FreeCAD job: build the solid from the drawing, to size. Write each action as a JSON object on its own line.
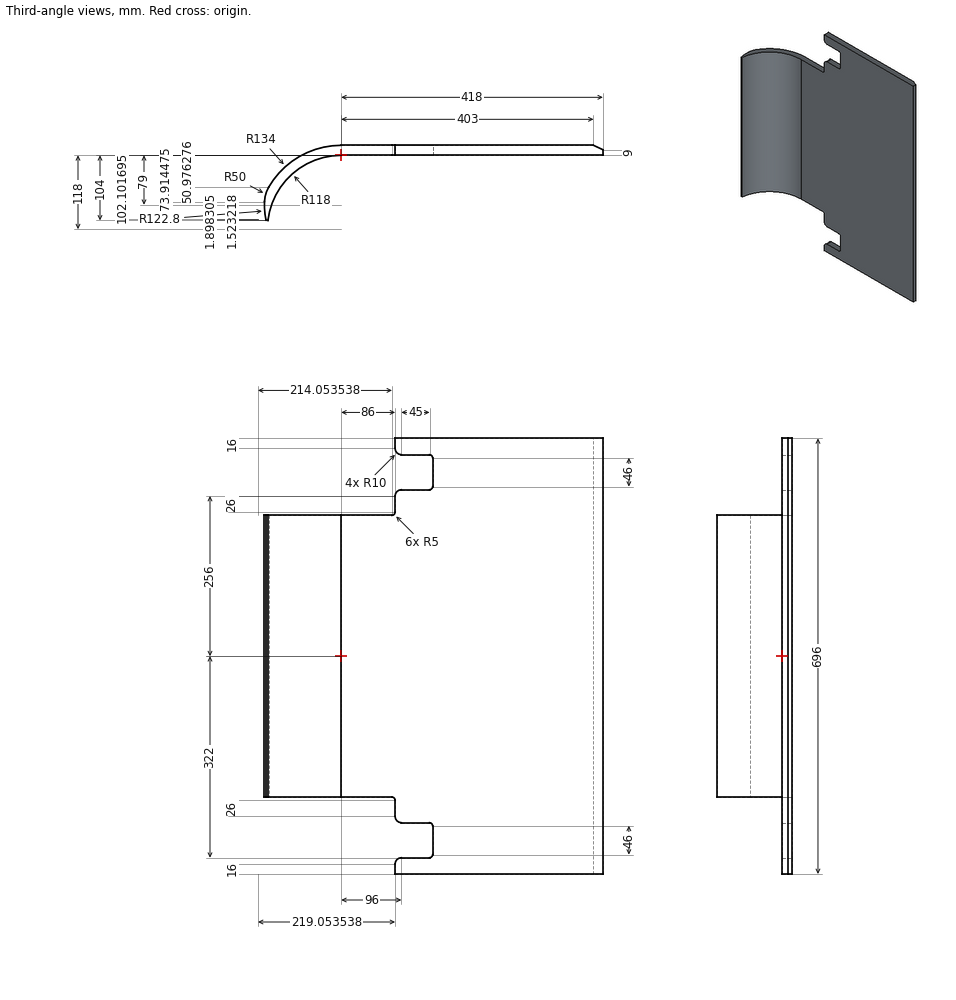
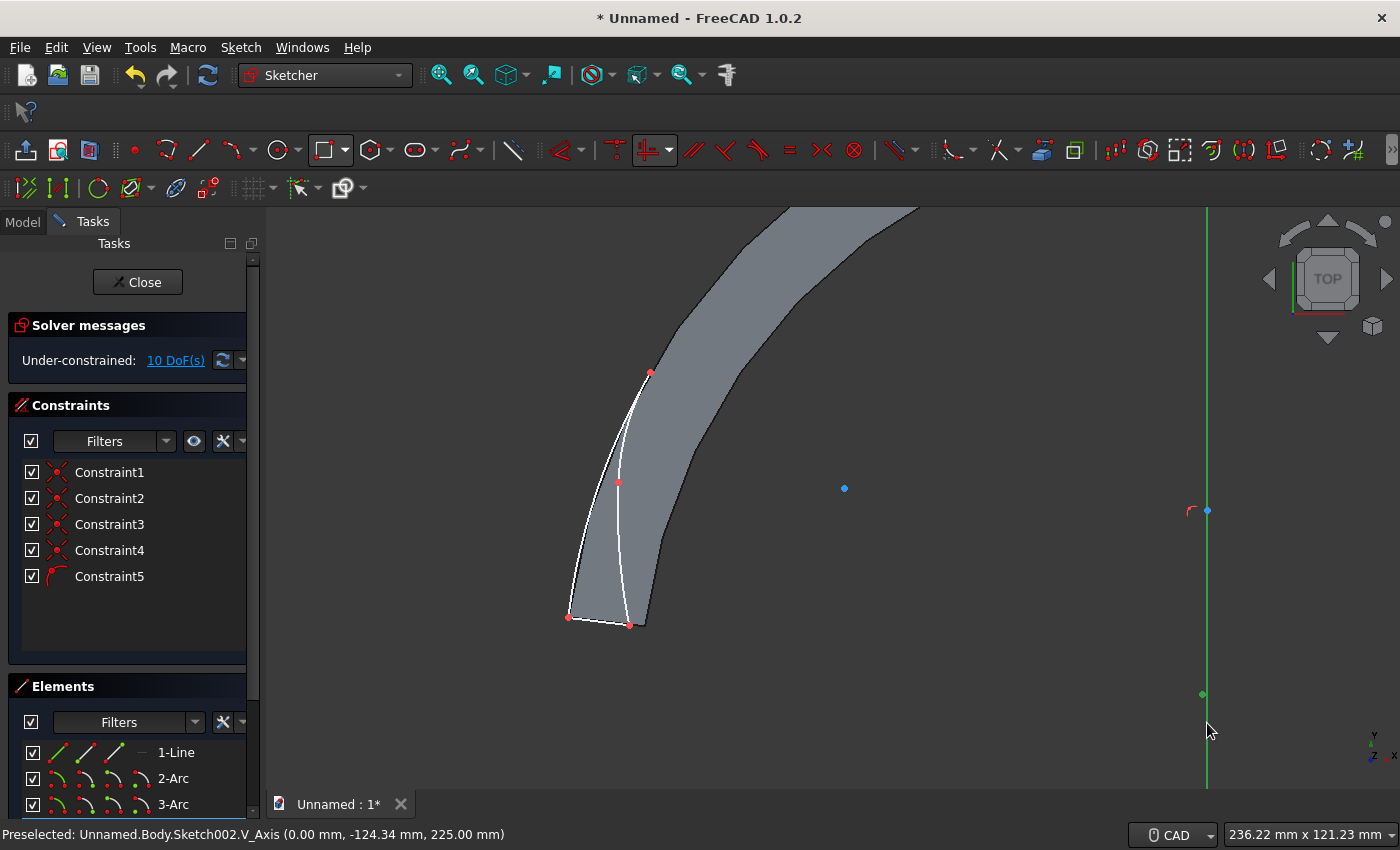
{"action": "left_click", "coordinate": [616, 150]}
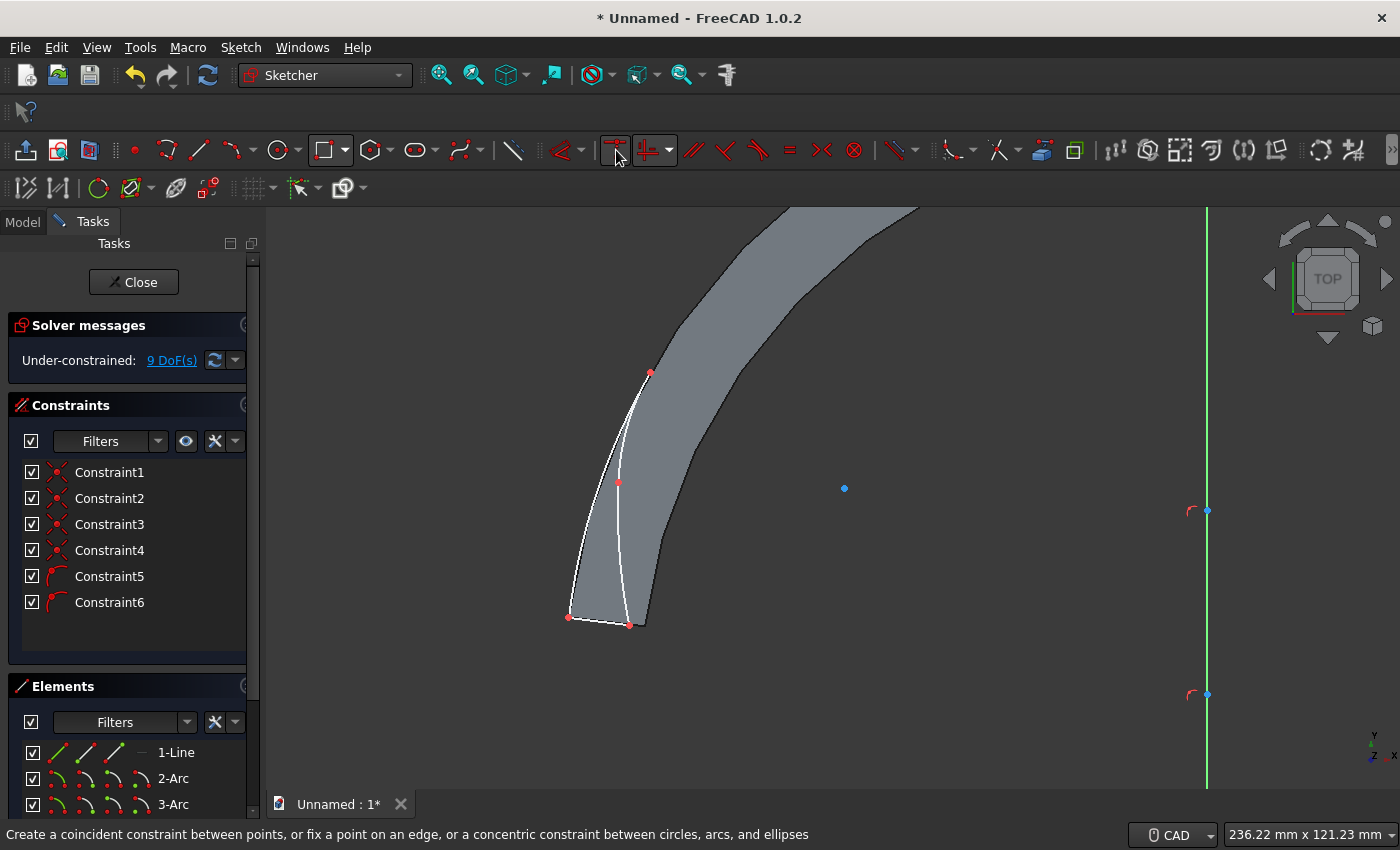
{"action": "left_click", "coordinate": [560, 150]}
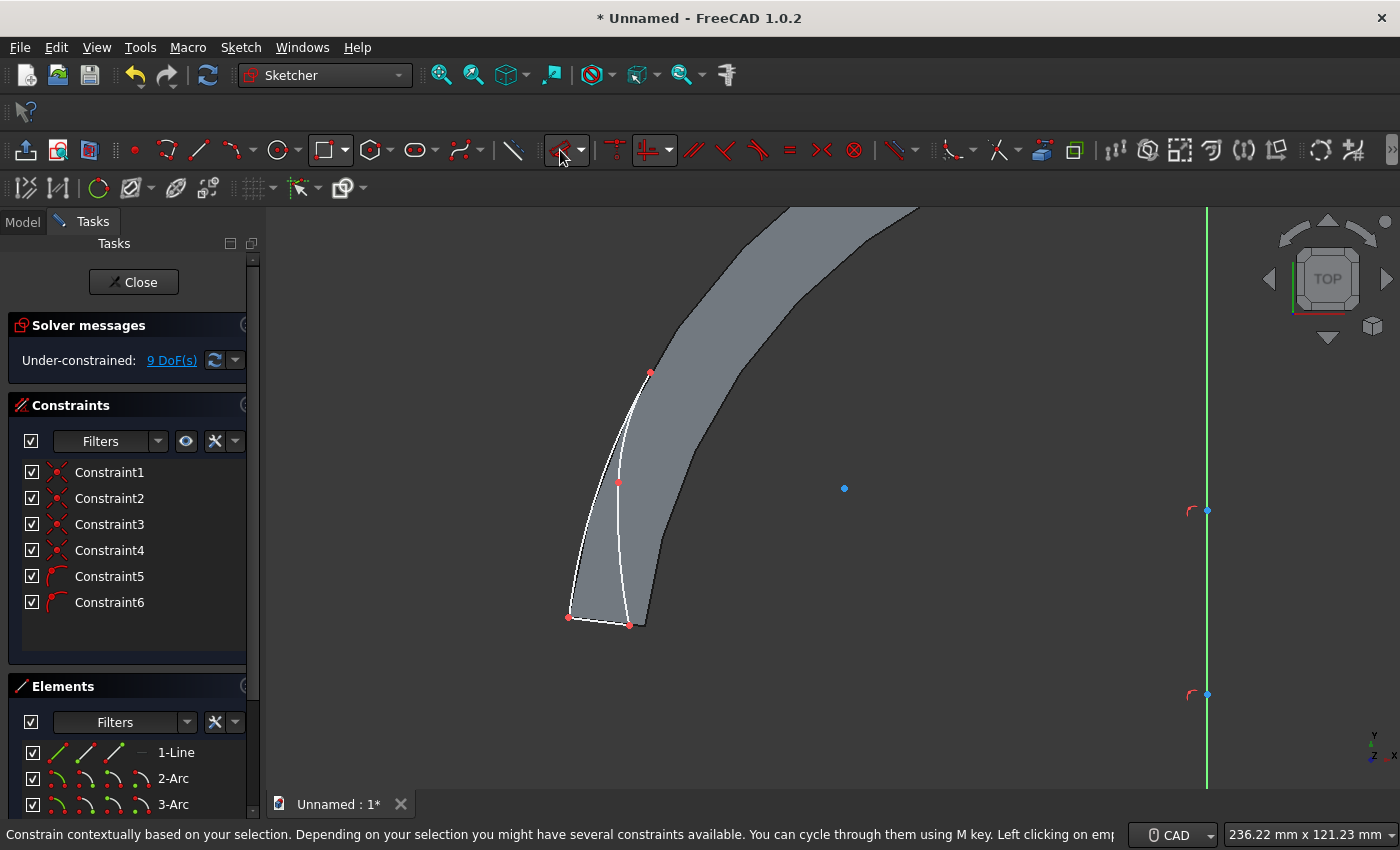
{"action": "left_click", "coordinate": [618, 526]}
{"action": "left_click", "coordinate": [563, 527]}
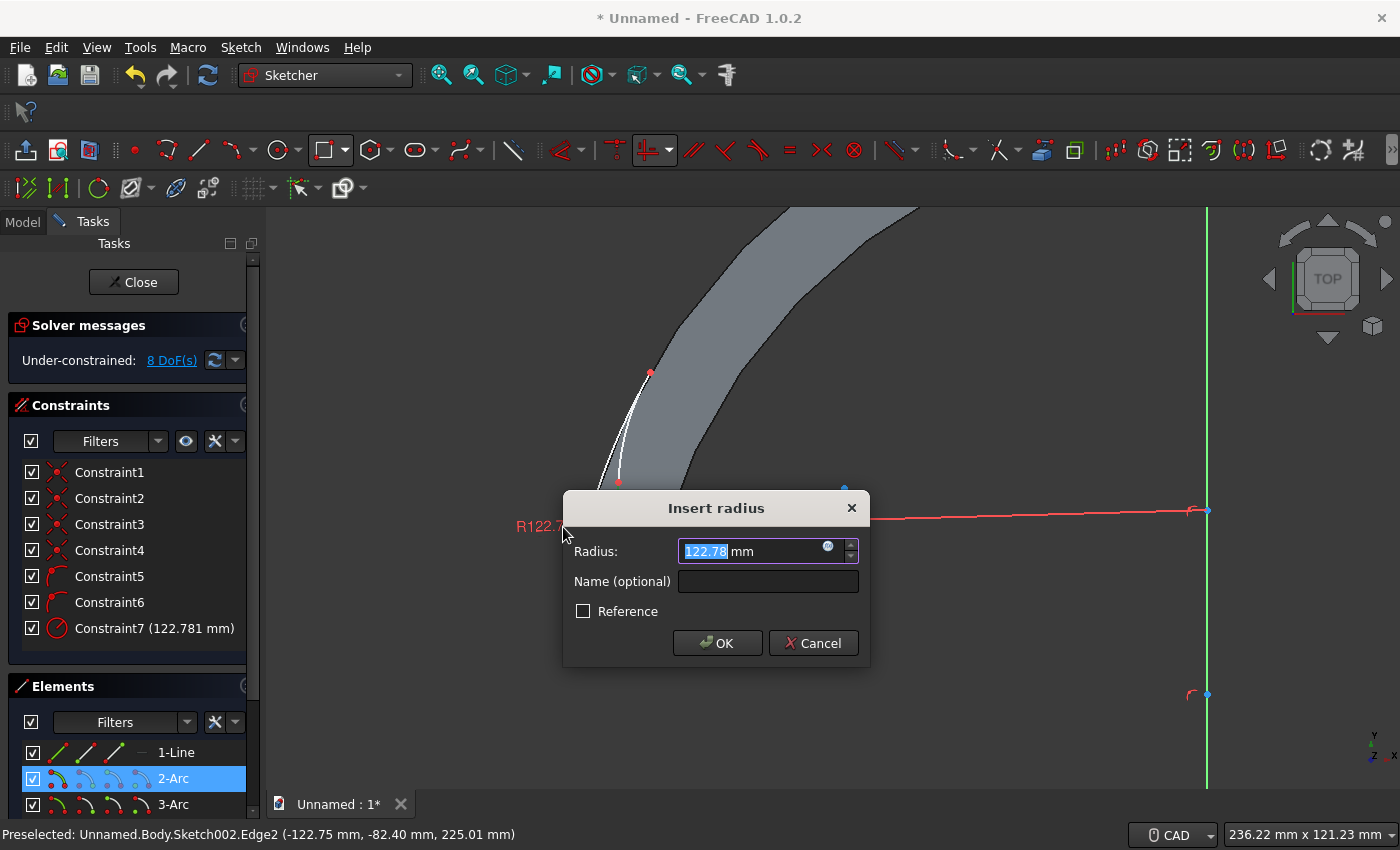
{"action": "type", "text": "122.8"}
{"action": "key", "text": "Return"}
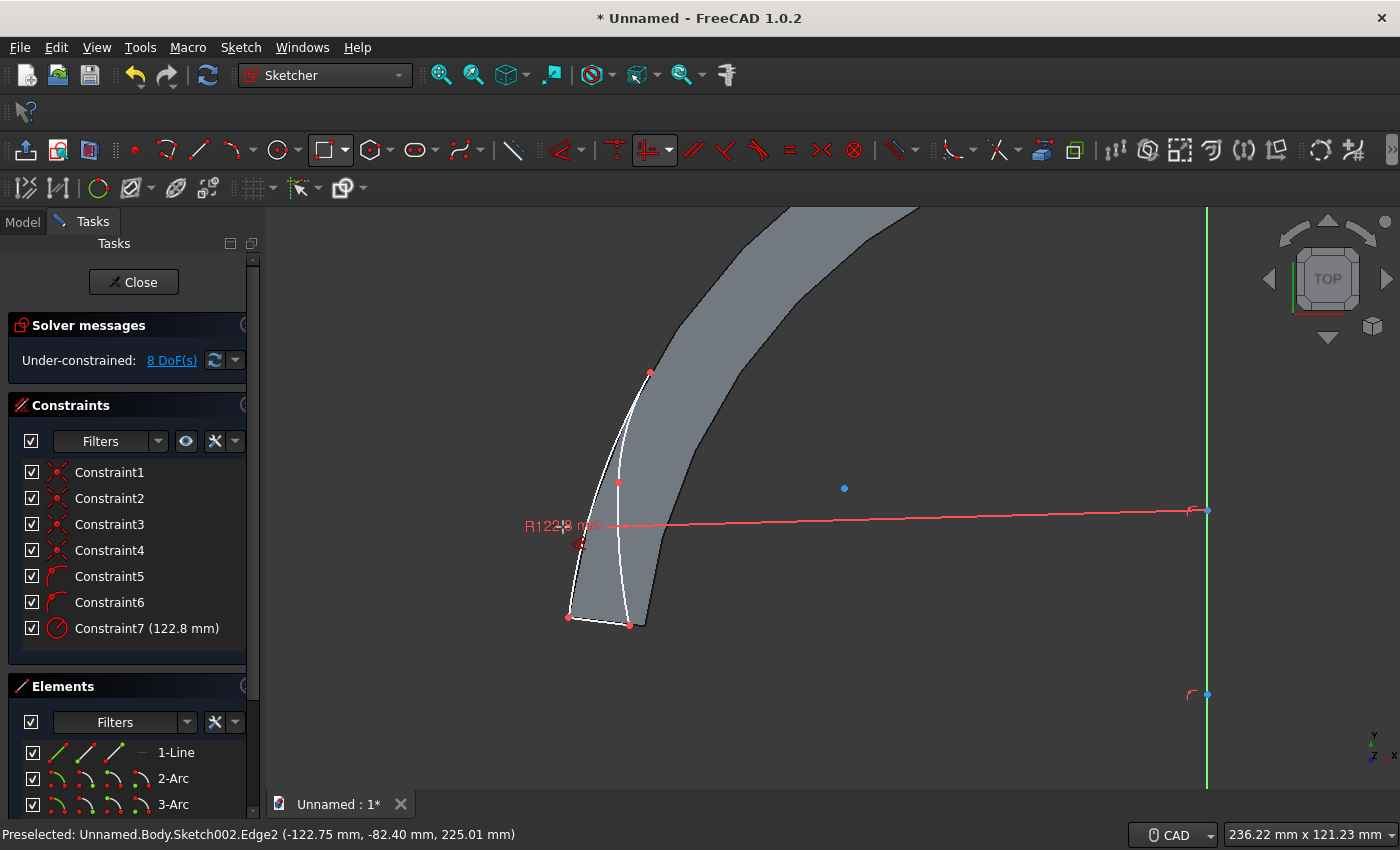
{"action": "scroll", "coordinate": [620, 459], "scroll_direction": "up", "scroll_amount": 2}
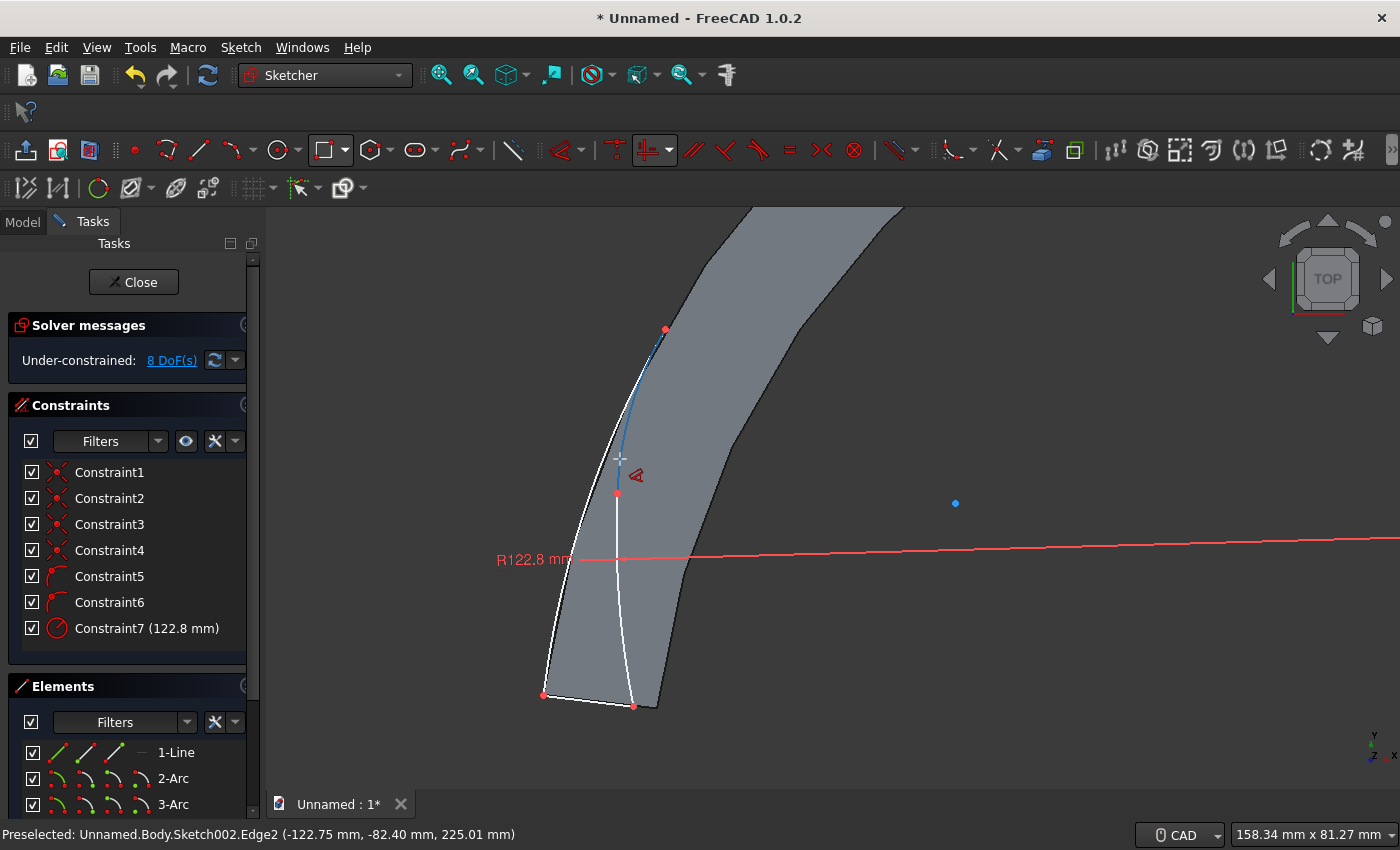
{"action": "left_click", "coordinate": [620, 459]}
{"action": "left_click", "coordinate": [588, 455]}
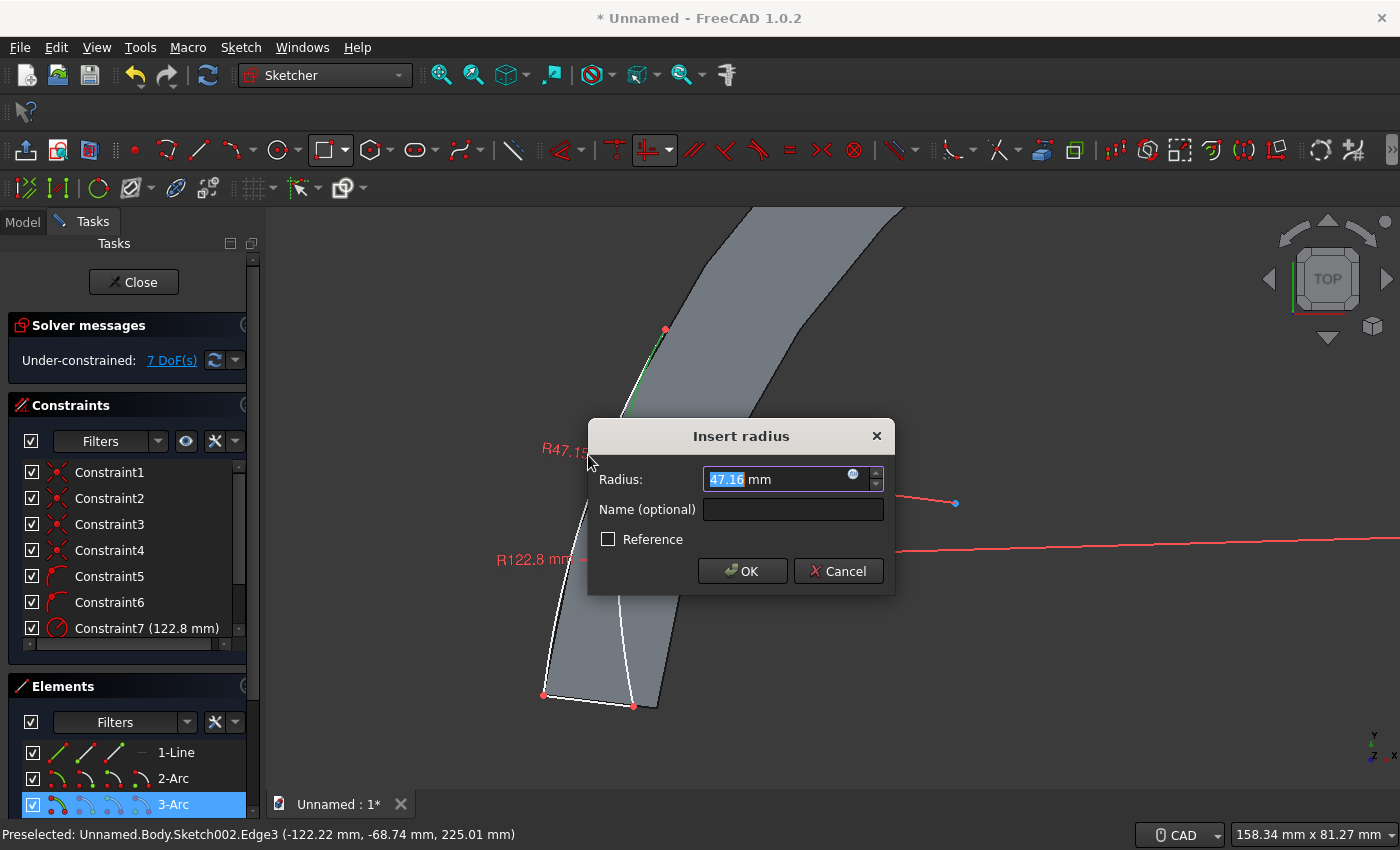
{"action": "type", "text": "50"}
{"action": "key", "text": "Return"}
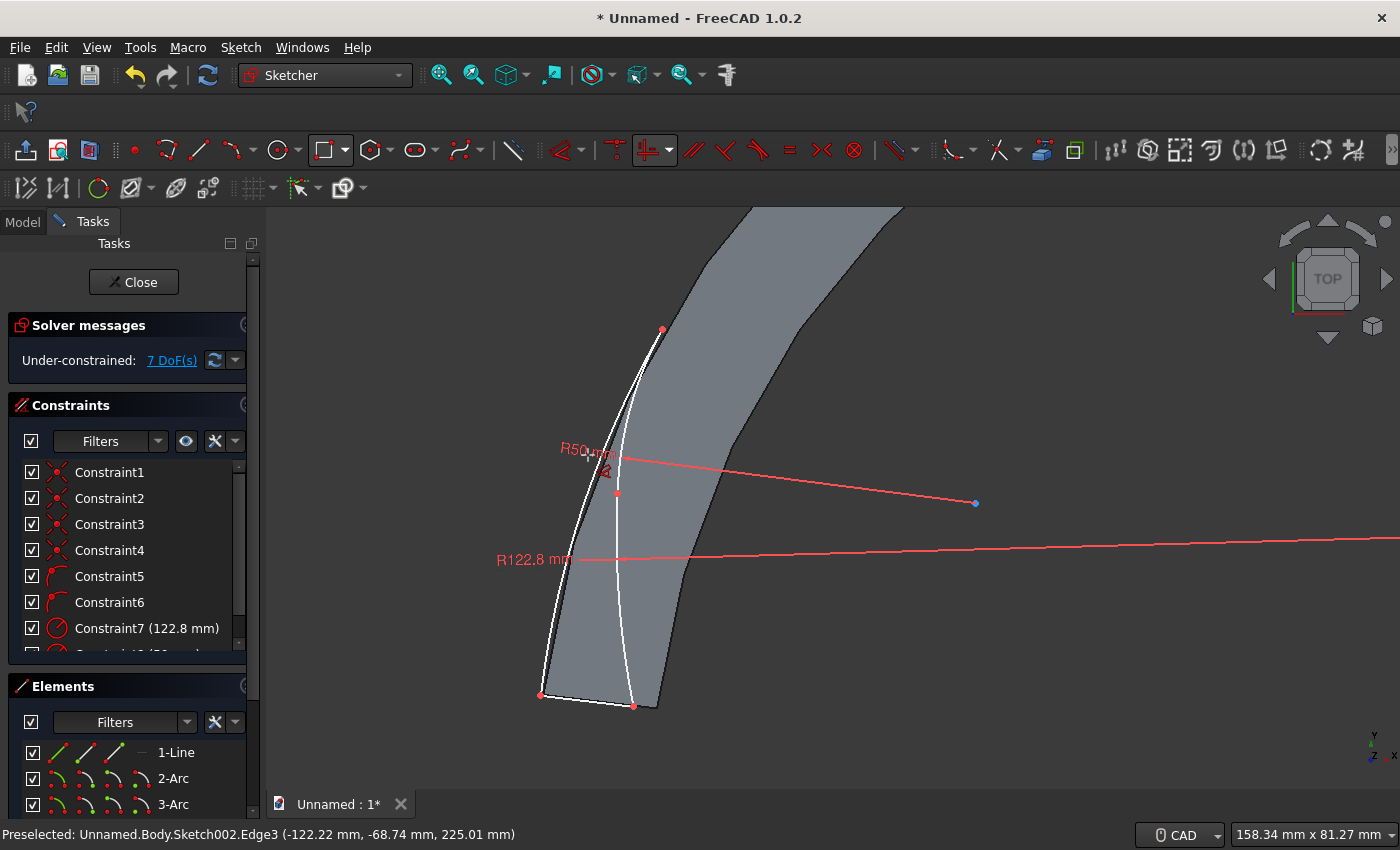
{"action": "left_click", "coordinate": [610, 434]}
{"action": "left_click", "coordinate": [581, 422]}